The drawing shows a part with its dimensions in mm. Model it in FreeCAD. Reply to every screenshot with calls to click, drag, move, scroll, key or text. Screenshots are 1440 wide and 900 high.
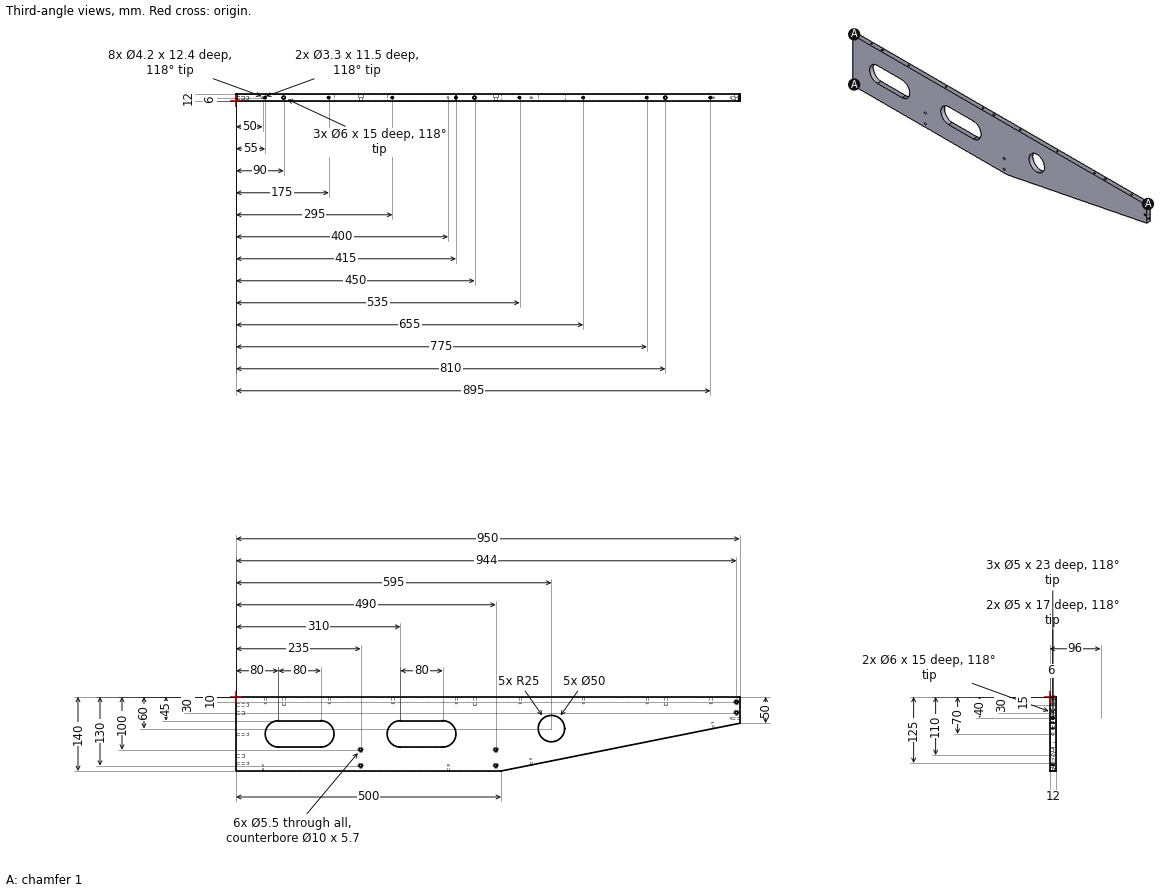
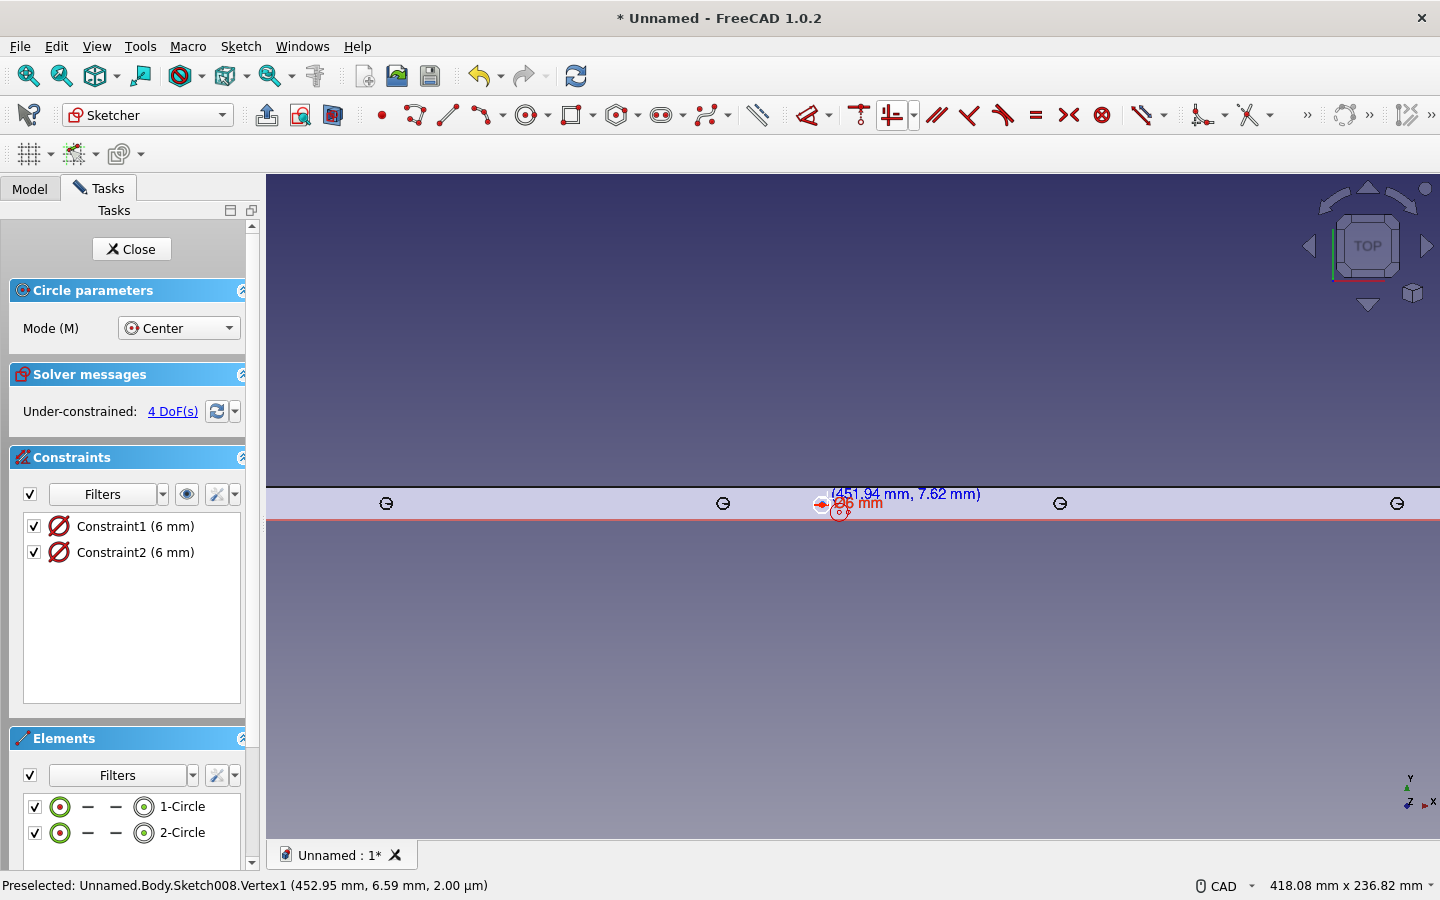
scroll(821, 506, down, 6)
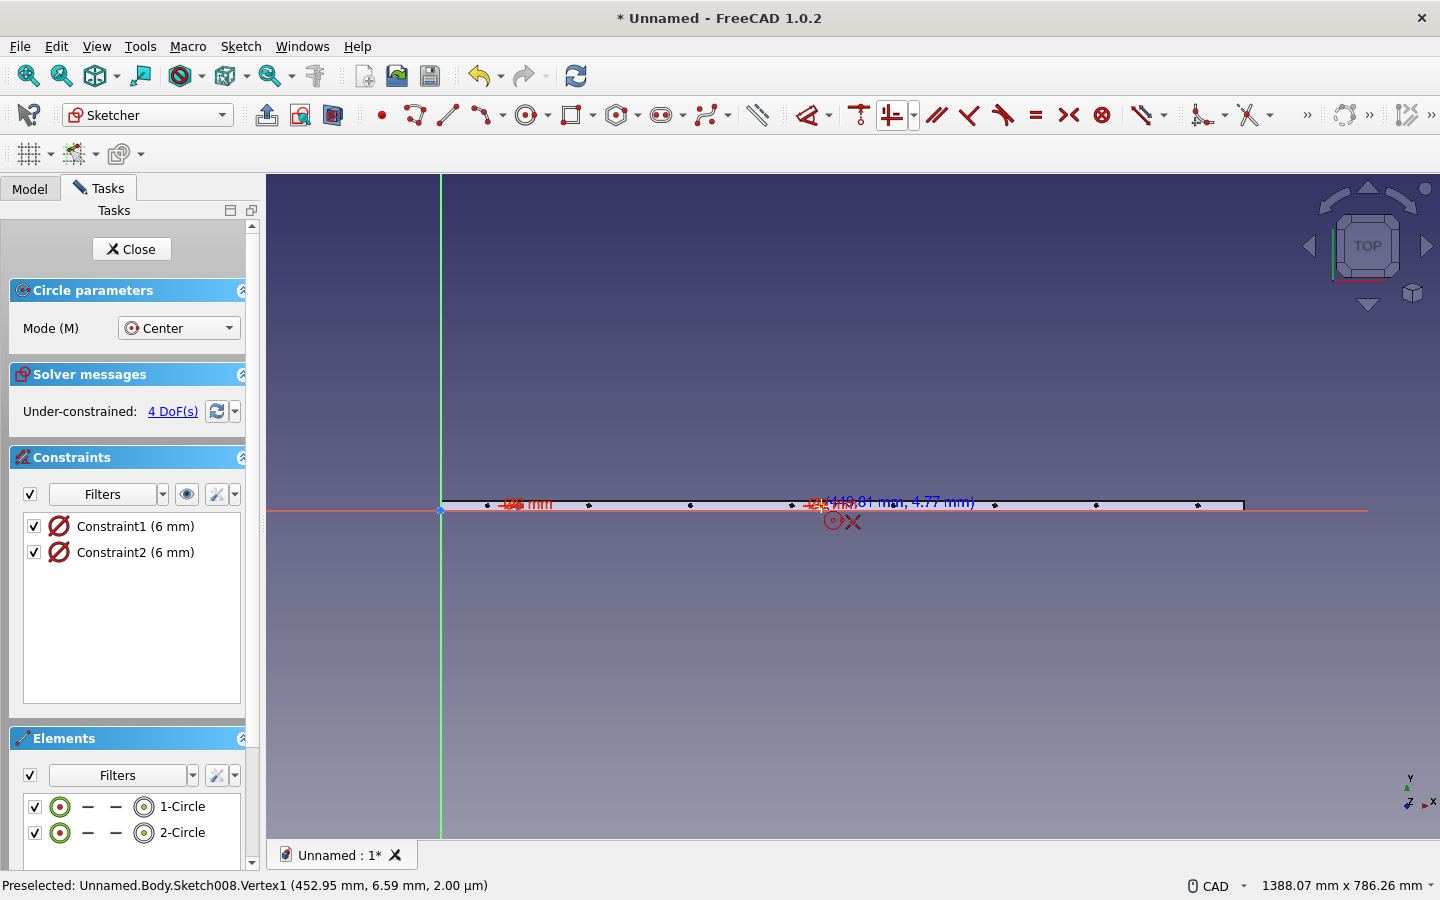
scroll(1126, 506, up, 11)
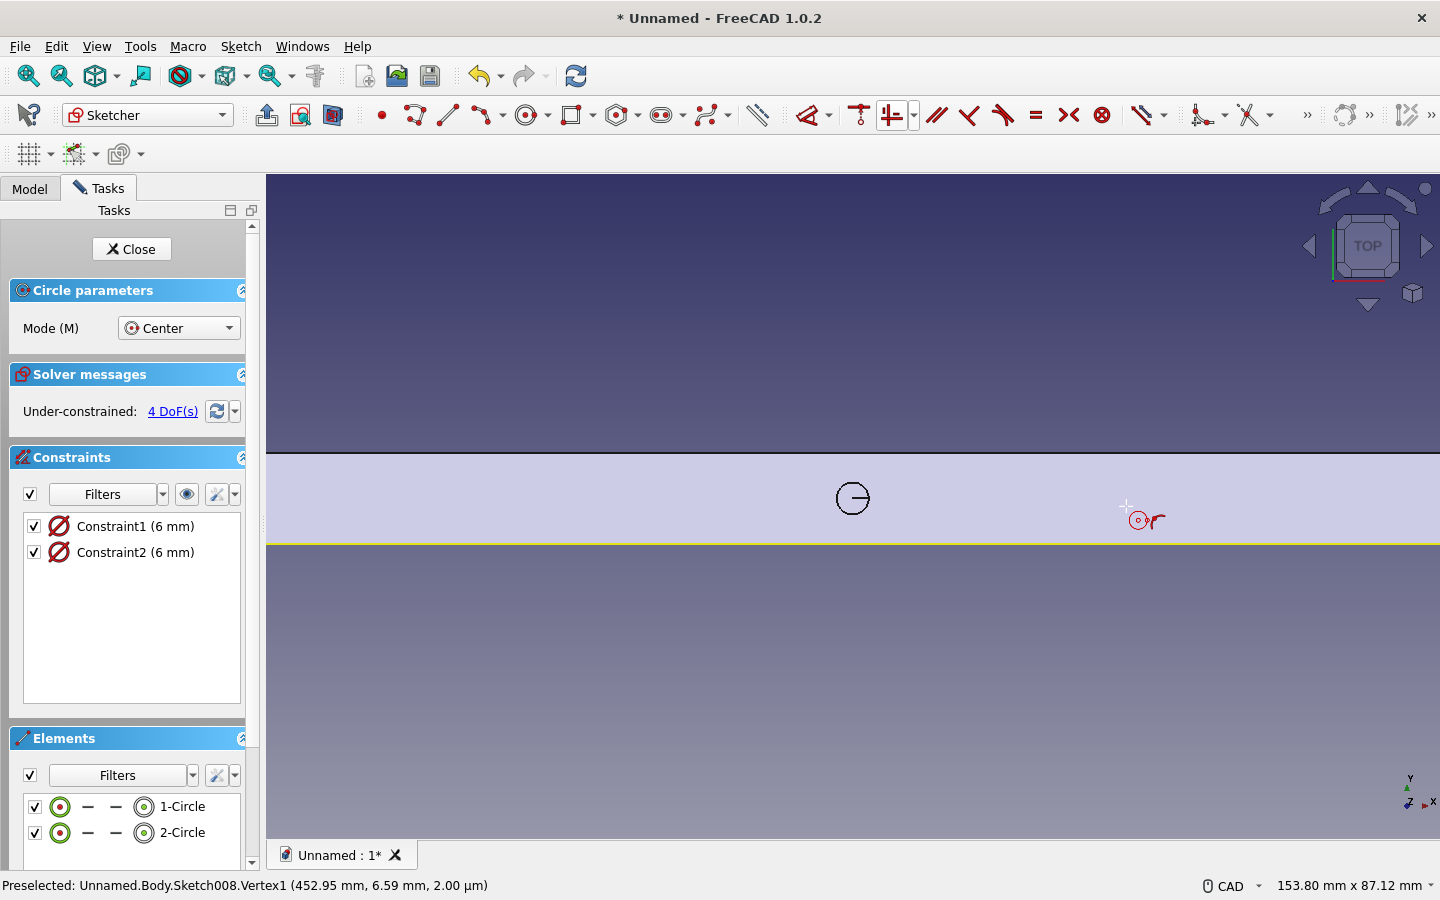
scroll(1127, 506, down, 11)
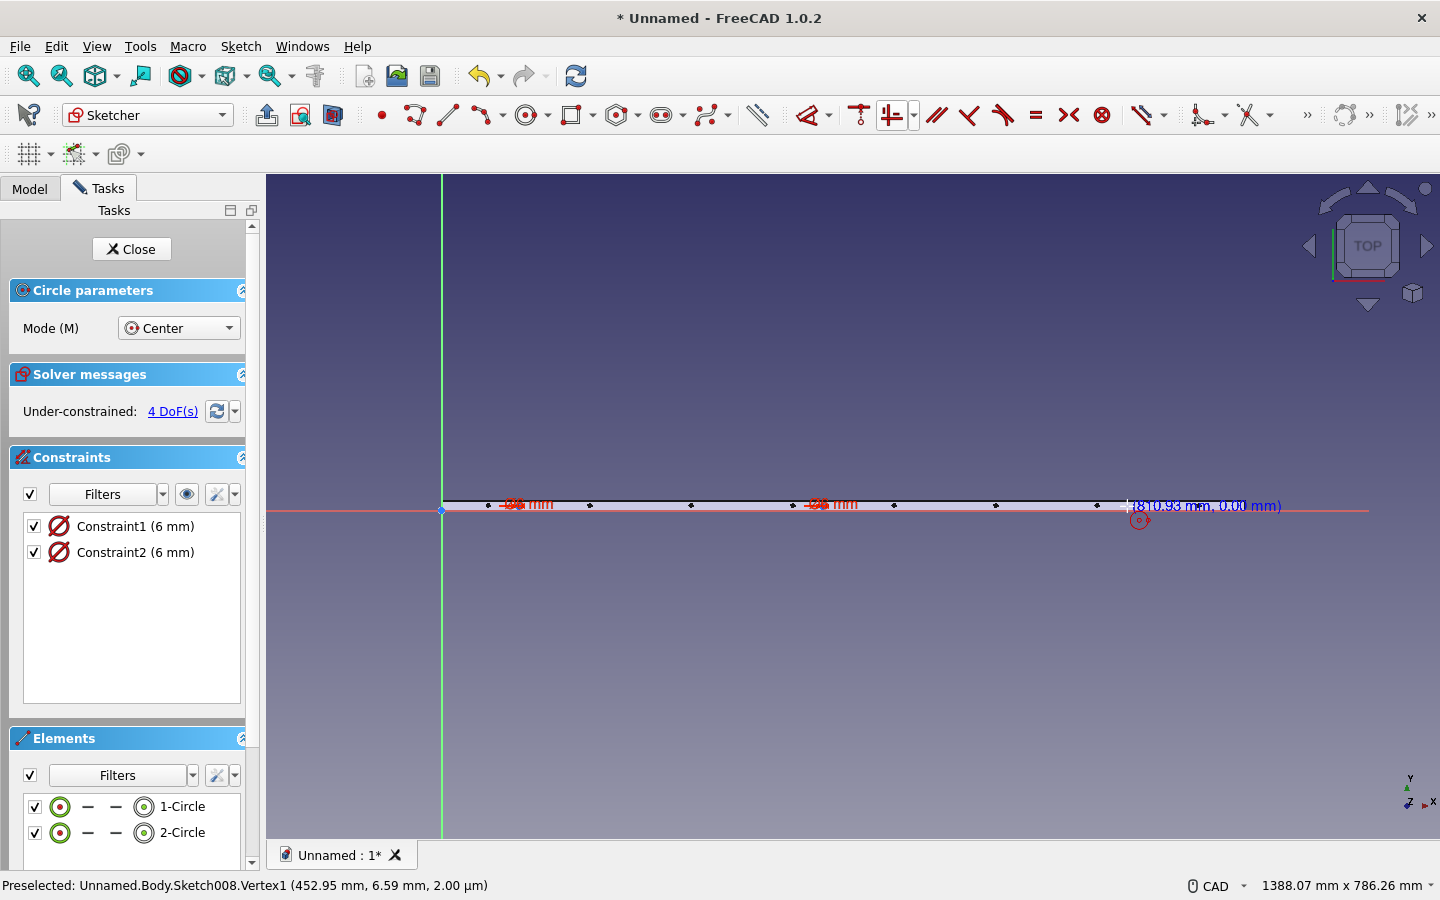
scroll(1127, 506, up, 6)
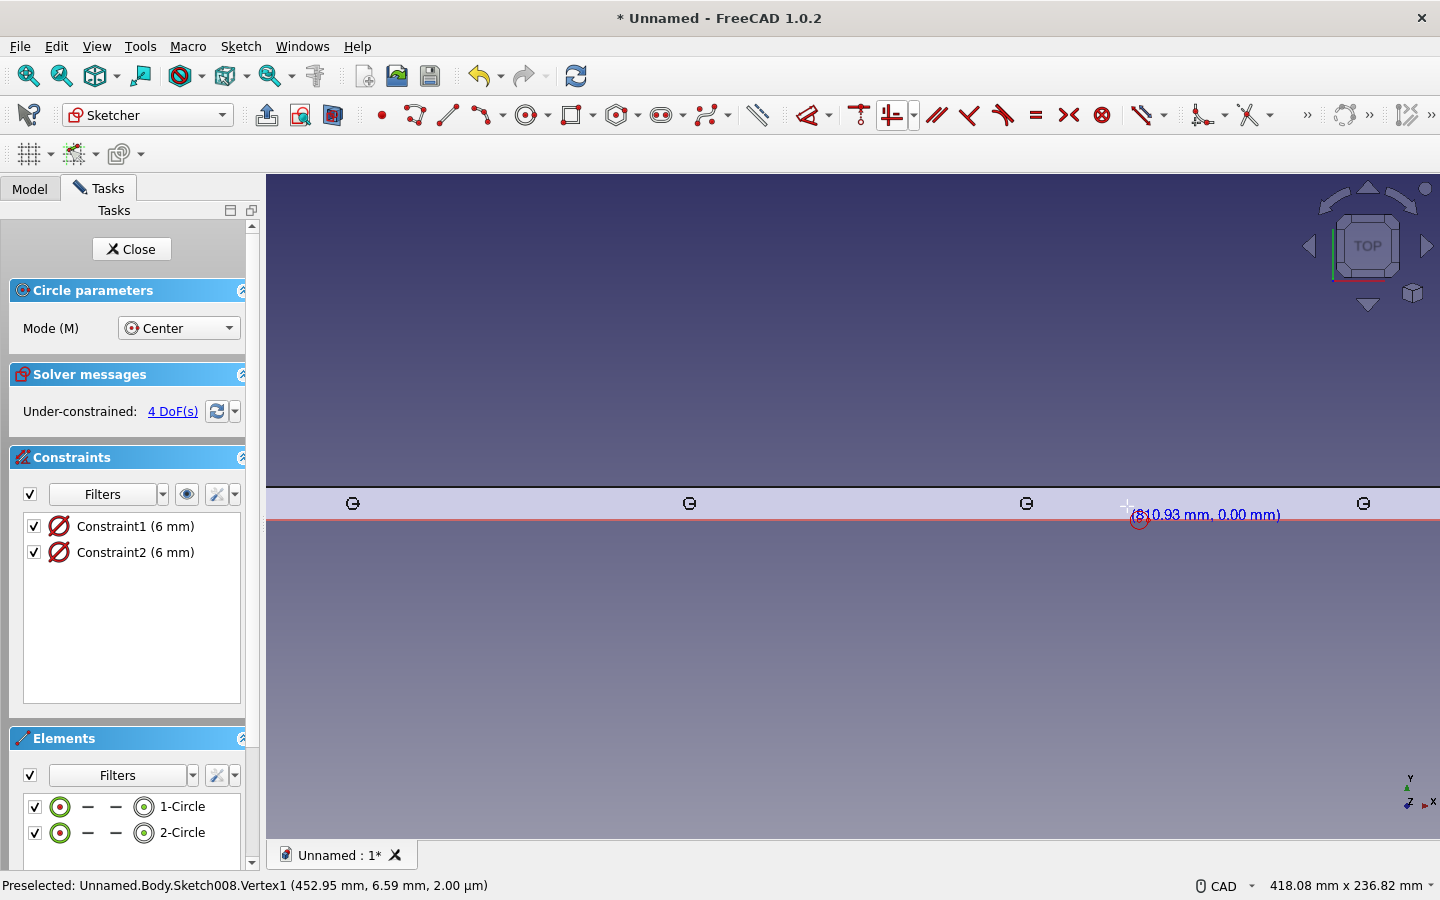
click(1125, 504)
move(1131, 498)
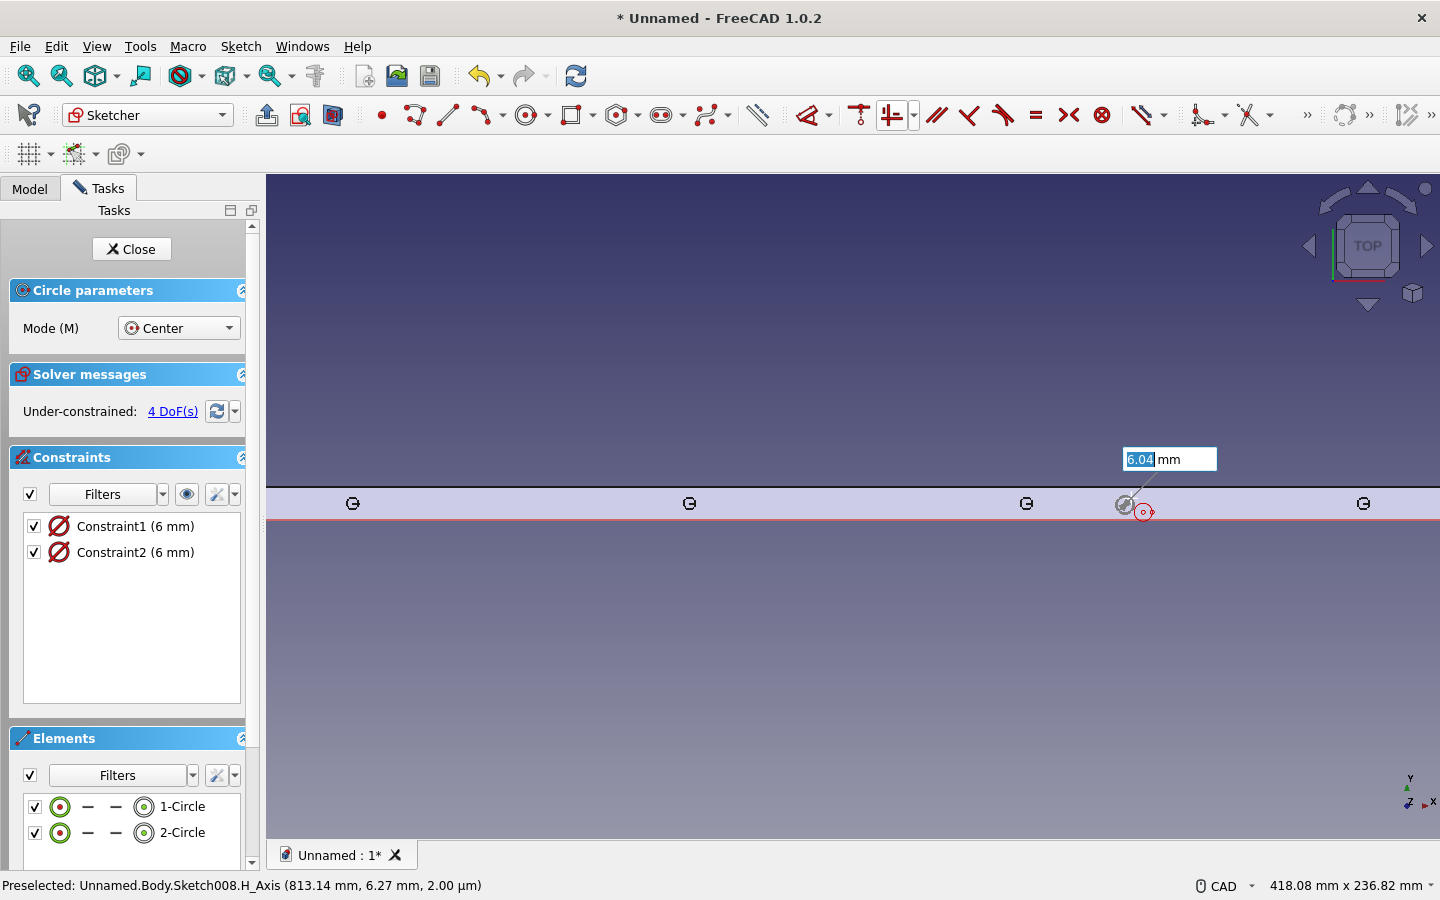
text(6)
key(Return)
key(Escape)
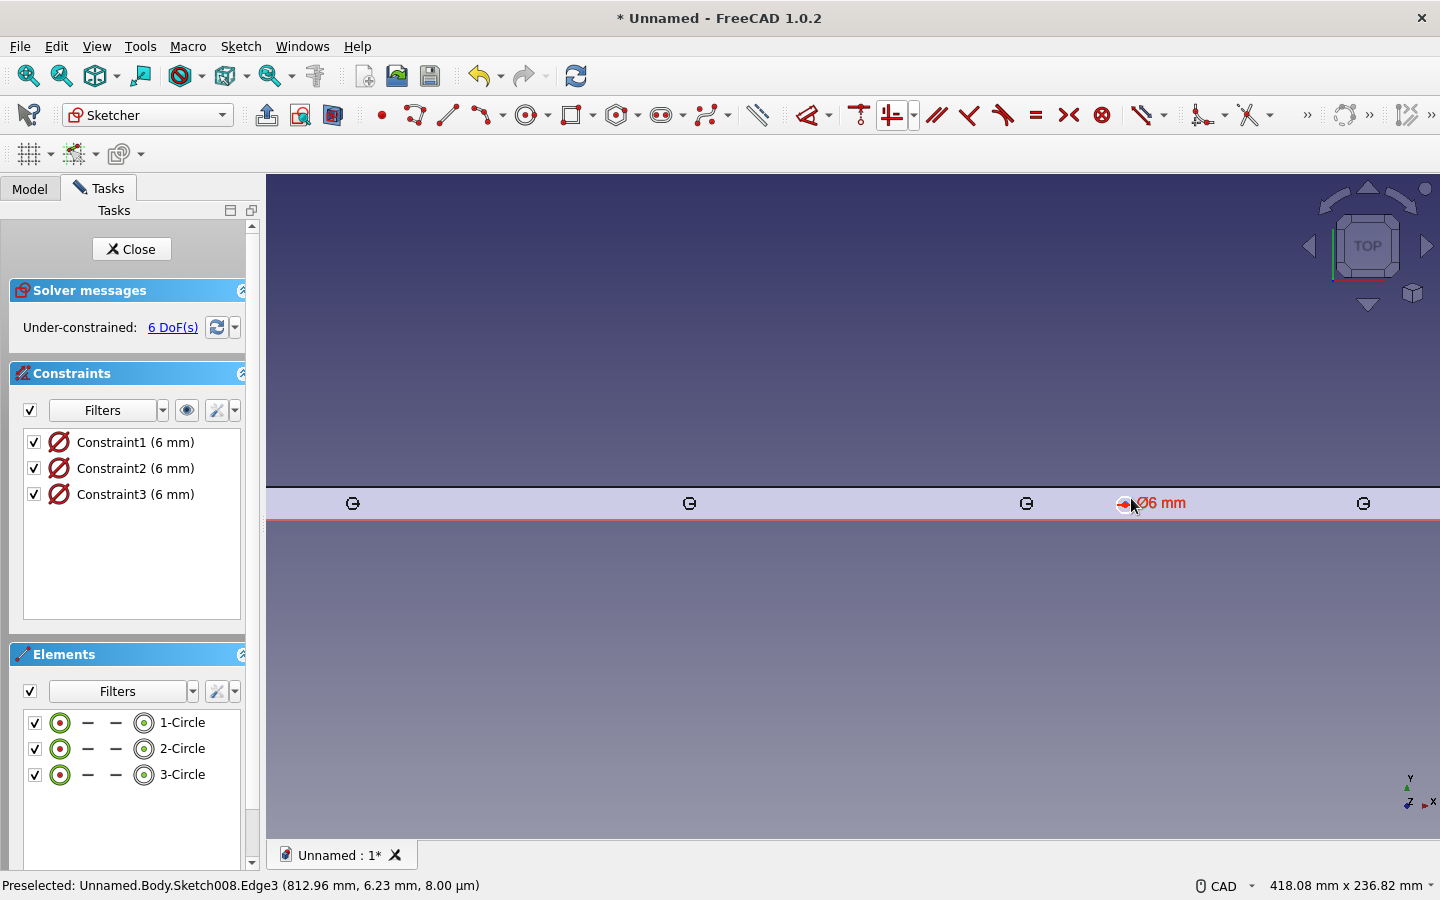
click(806, 116)